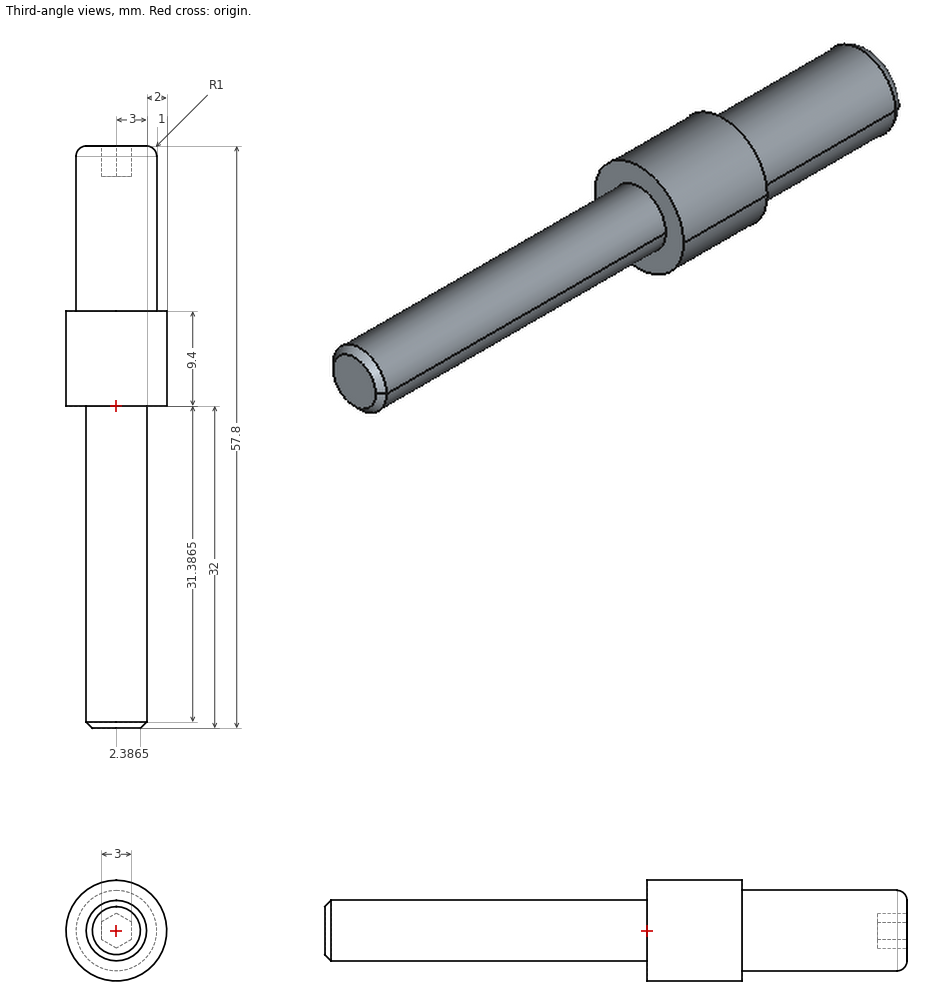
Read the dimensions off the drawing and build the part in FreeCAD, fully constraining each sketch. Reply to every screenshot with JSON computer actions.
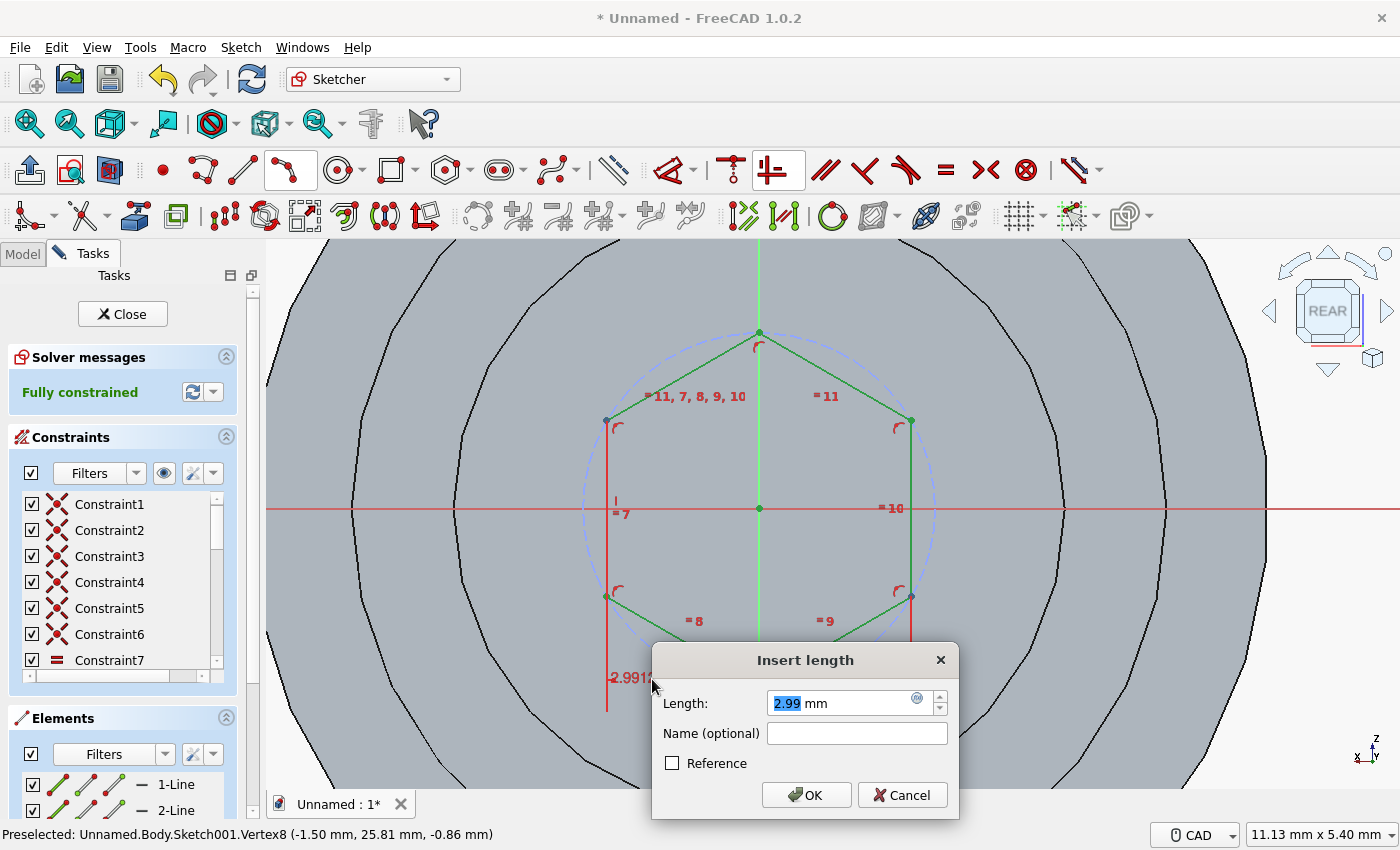
{"action": "type", "text": "3"}
{"action": "key", "text": "Return"}
{"action": "key", "text": "Escape"}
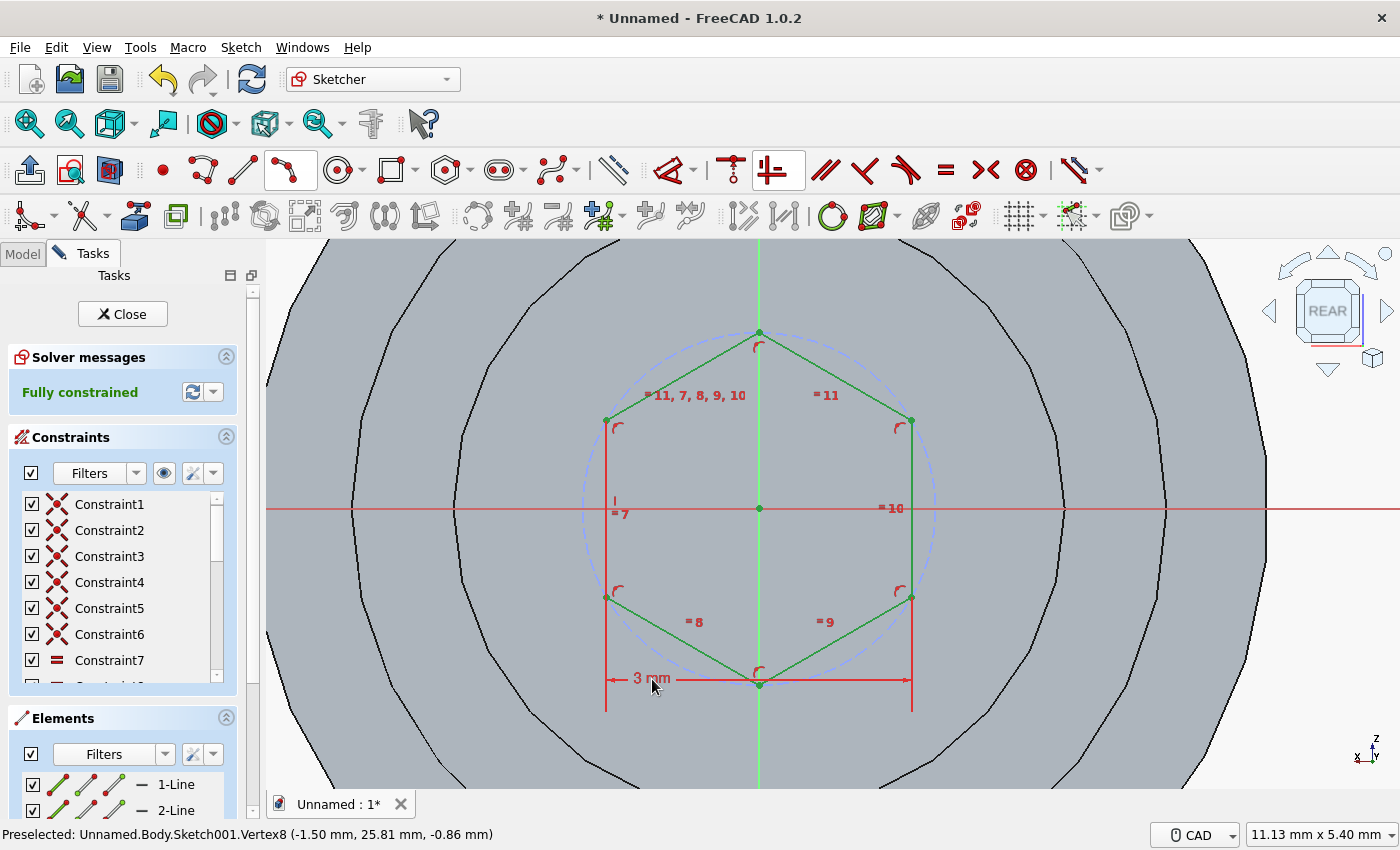
{"action": "left_click", "coordinate": [123, 314]}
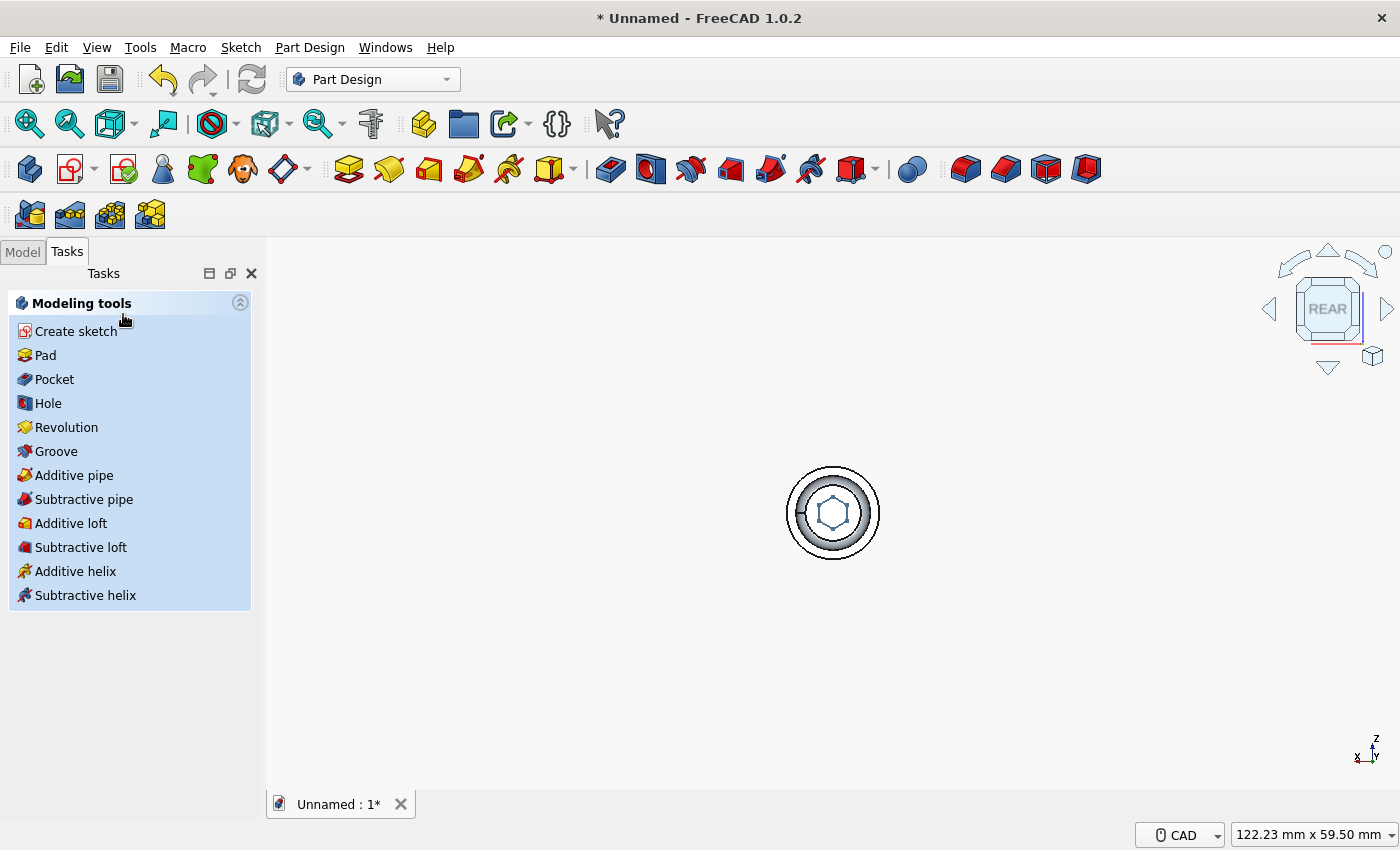
{"action": "left_click", "coordinate": [612, 170]}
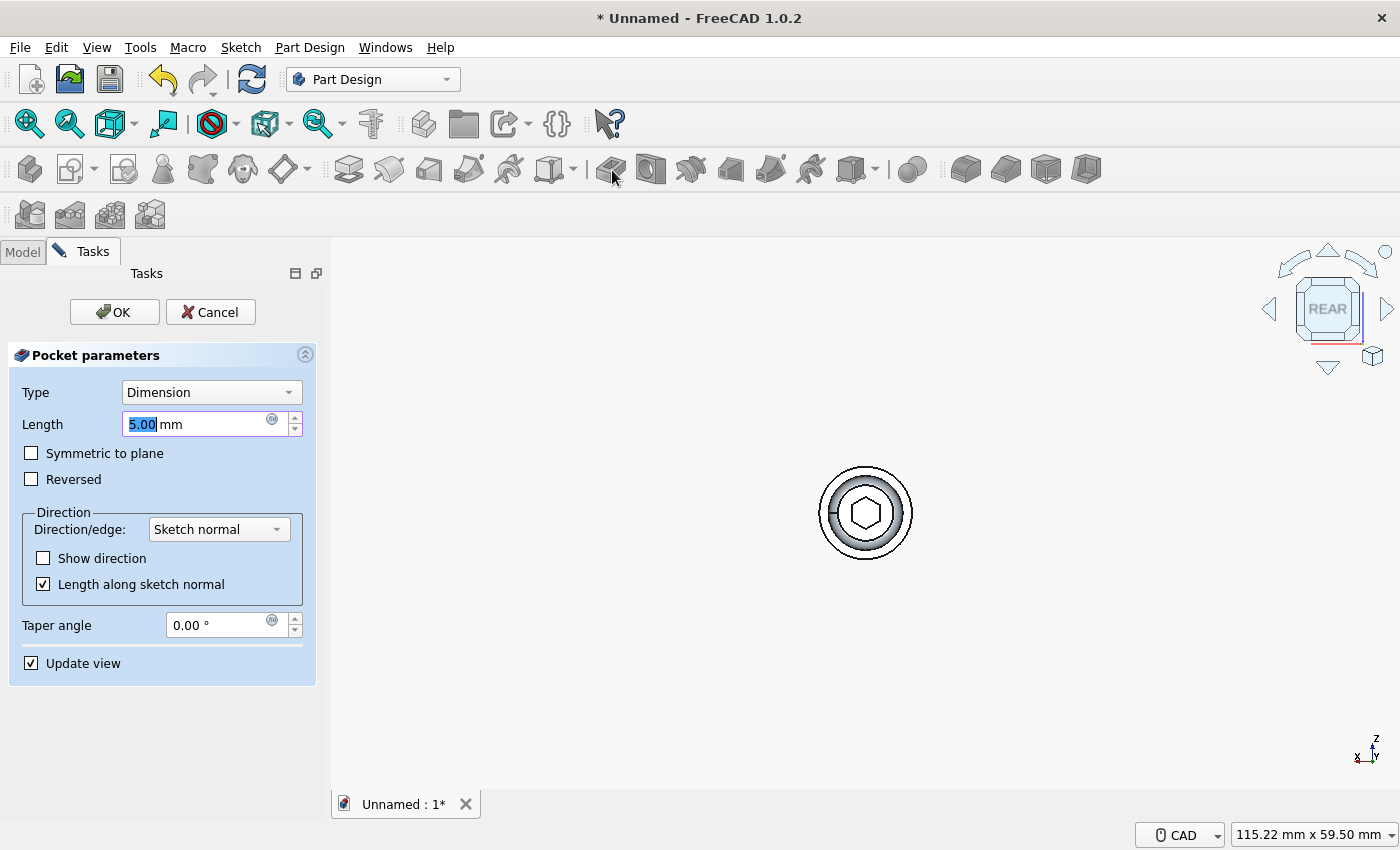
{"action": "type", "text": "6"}
{"action": "key", "text": "Tab"}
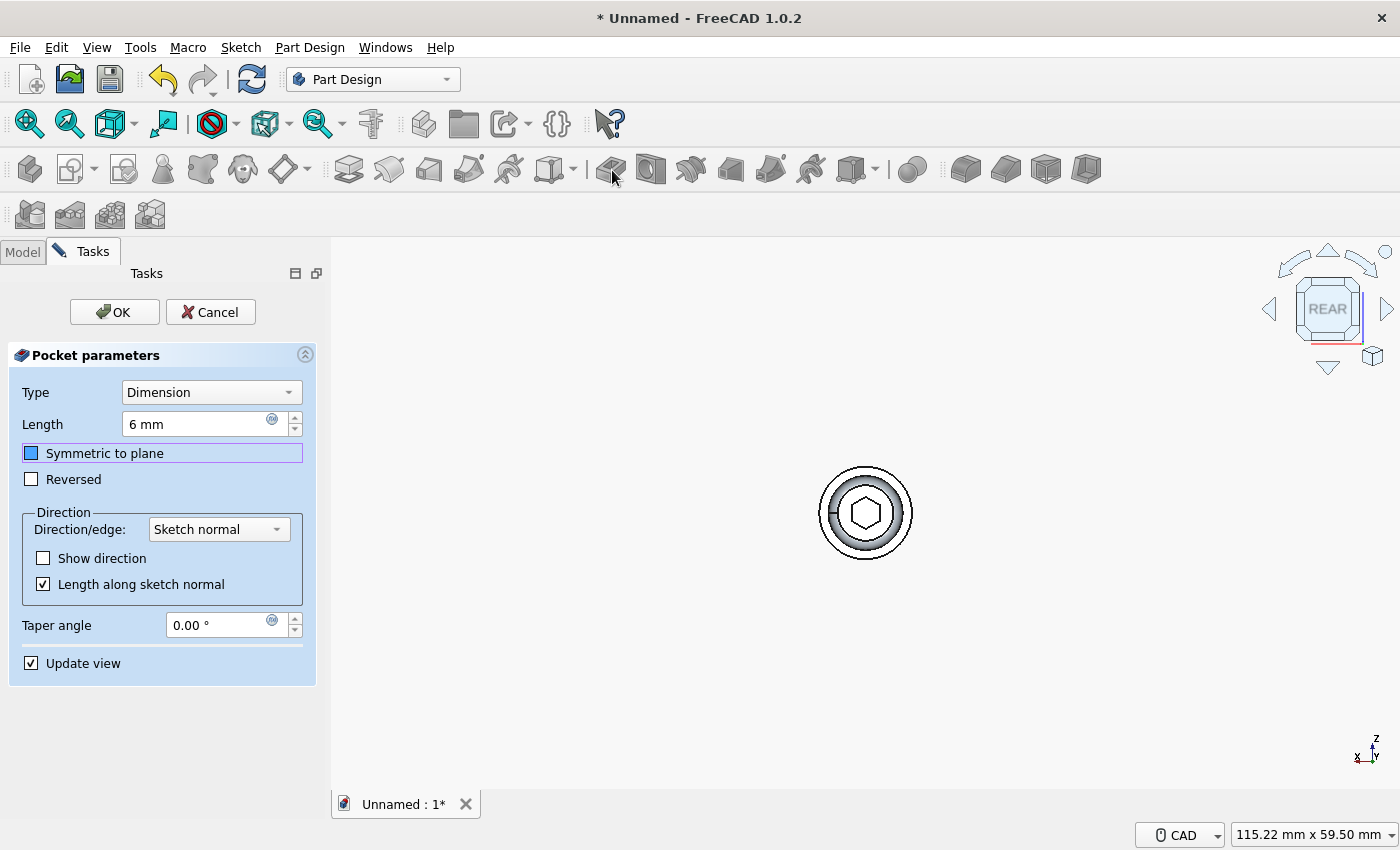
{"action": "left_click", "coordinate": [30, 453]}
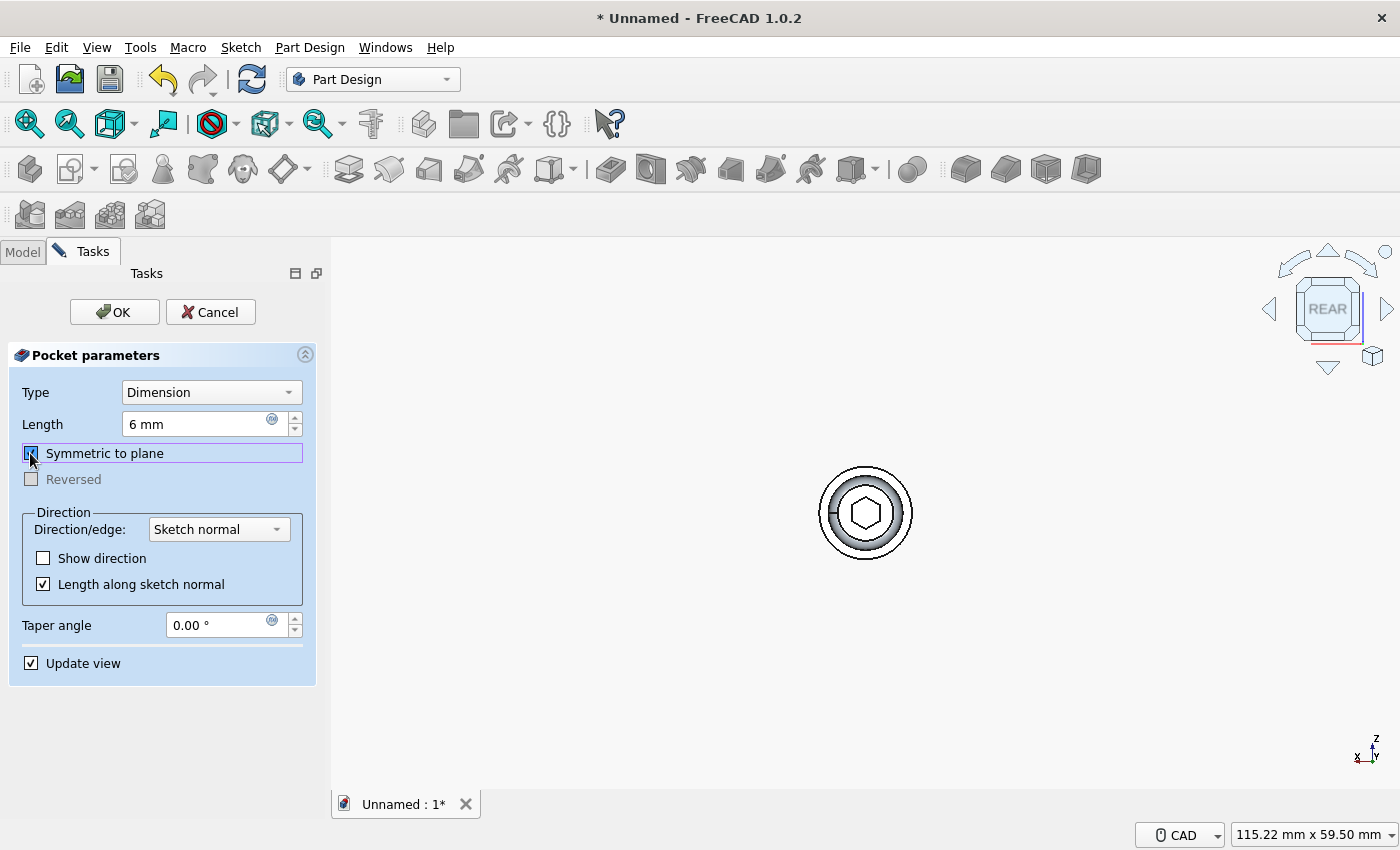
{"action": "left_click", "coordinate": [115, 312]}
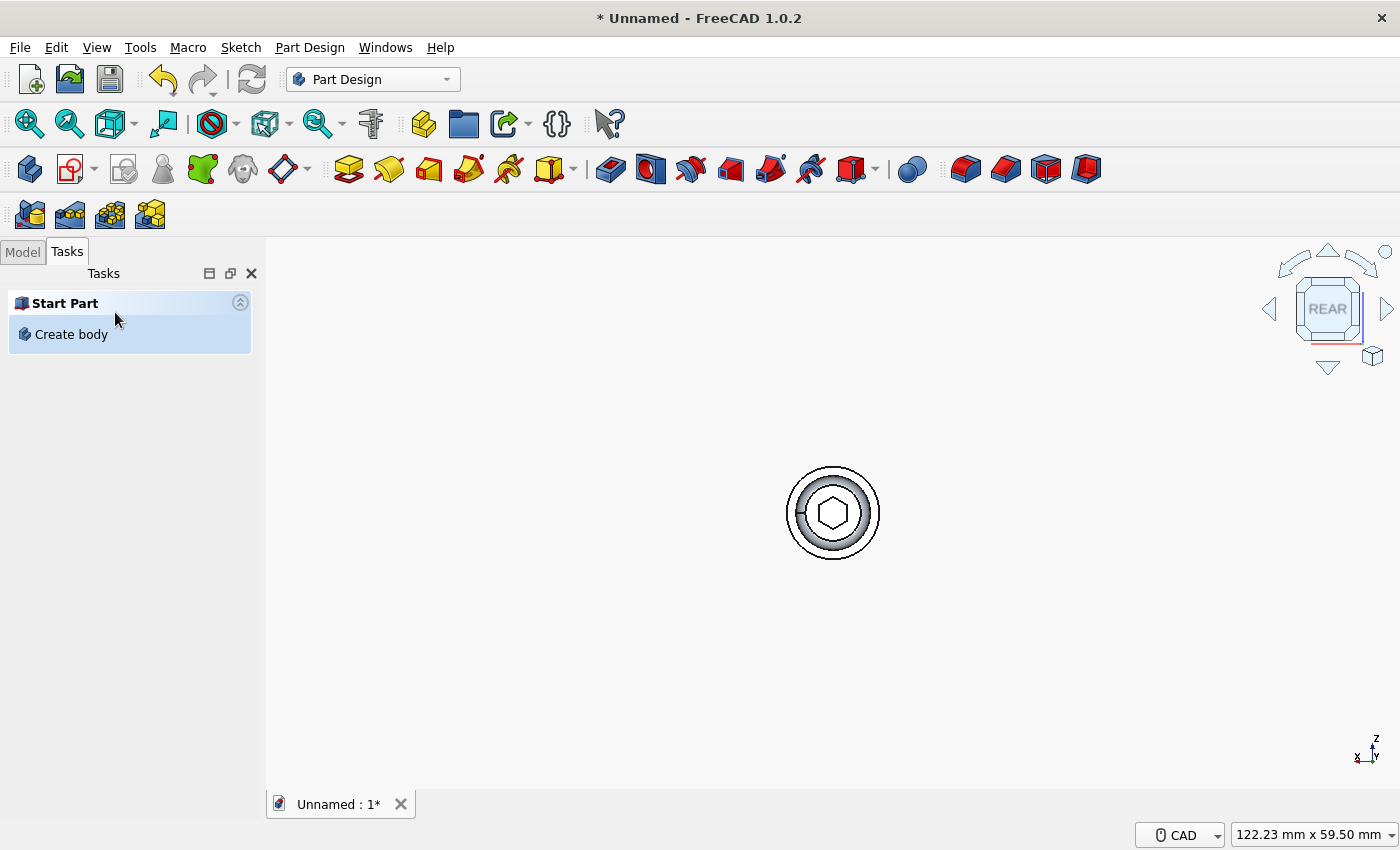
{"action": "key", "text": "0"}